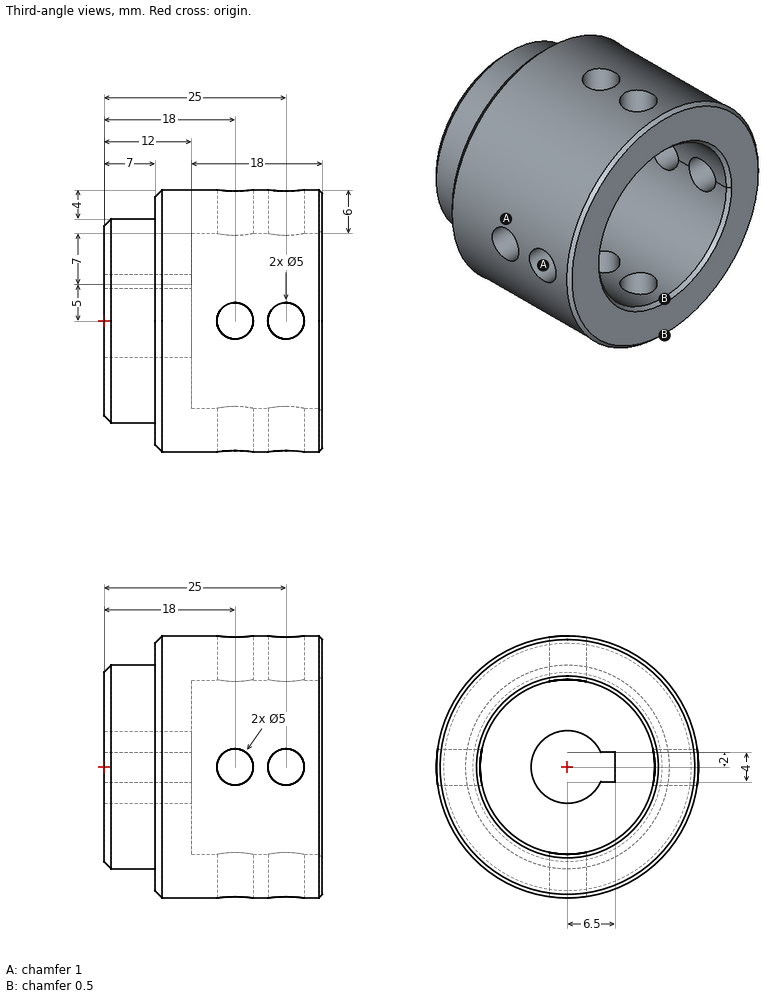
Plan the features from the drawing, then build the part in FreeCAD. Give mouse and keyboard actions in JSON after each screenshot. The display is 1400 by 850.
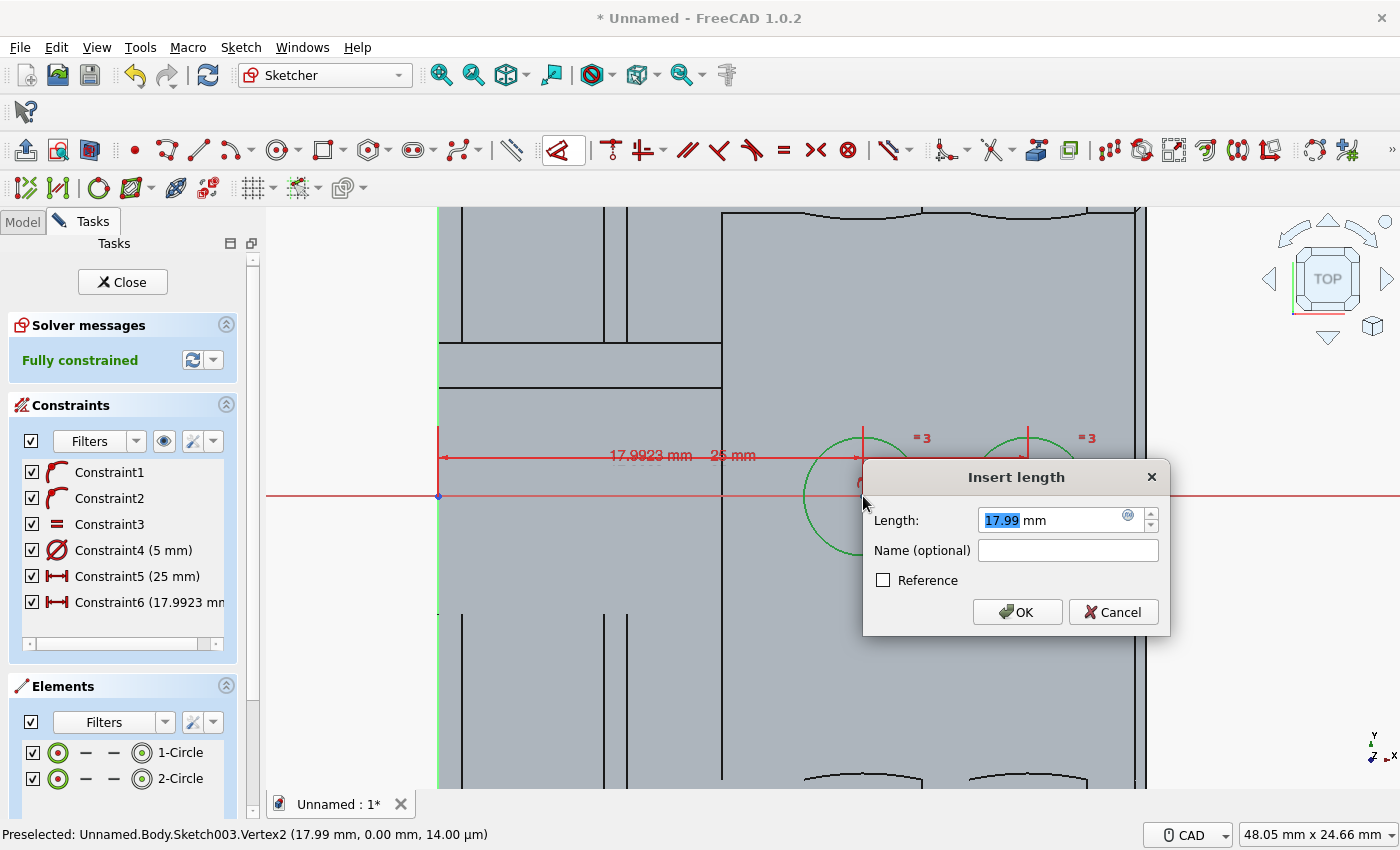
{"action": "type", "text": "18"}
{"action": "key", "text": "Return"}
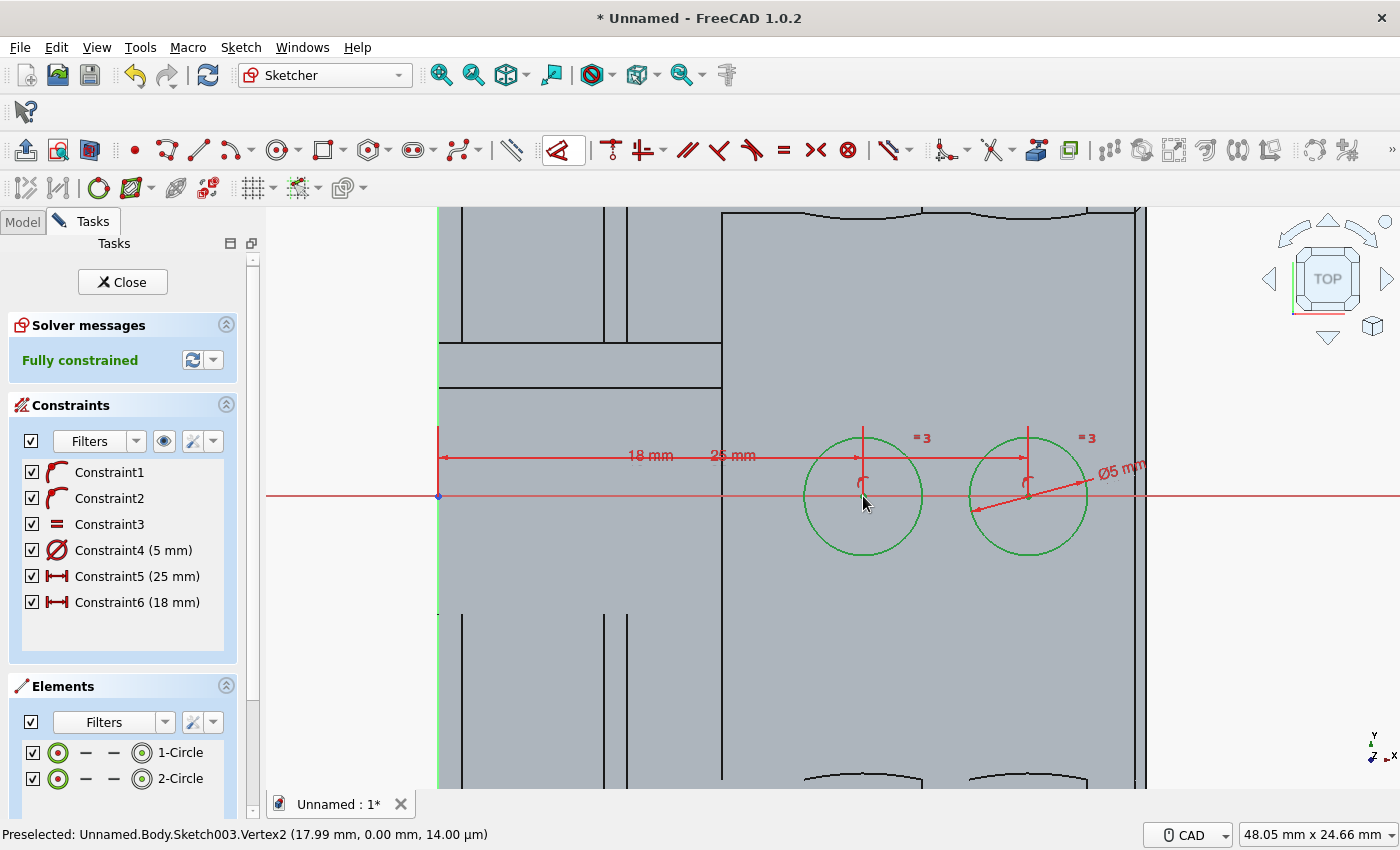
{"action": "left_click", "coordinate": [123, 282]}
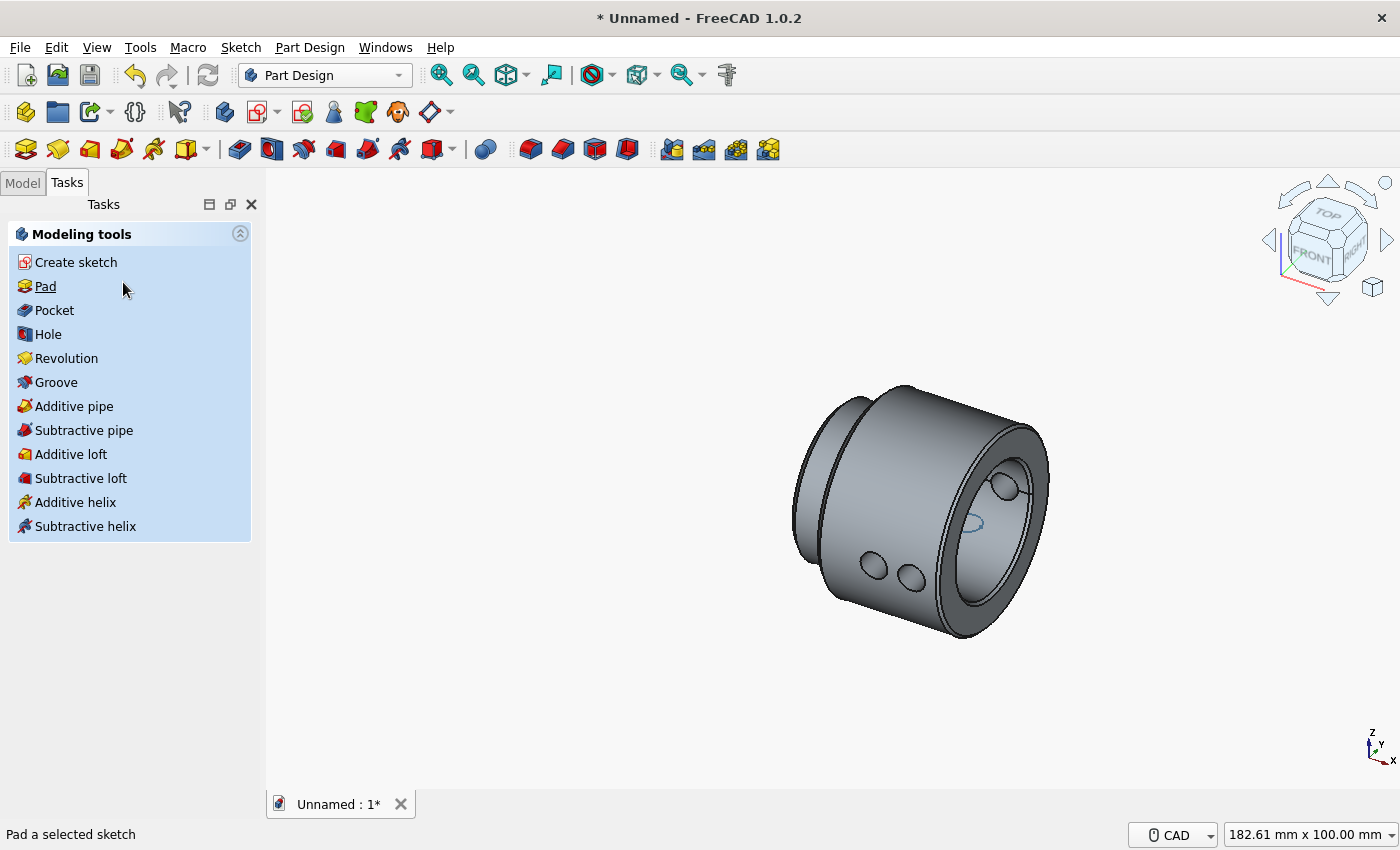
{"action": "left_click", "coordinate": [240, 150]}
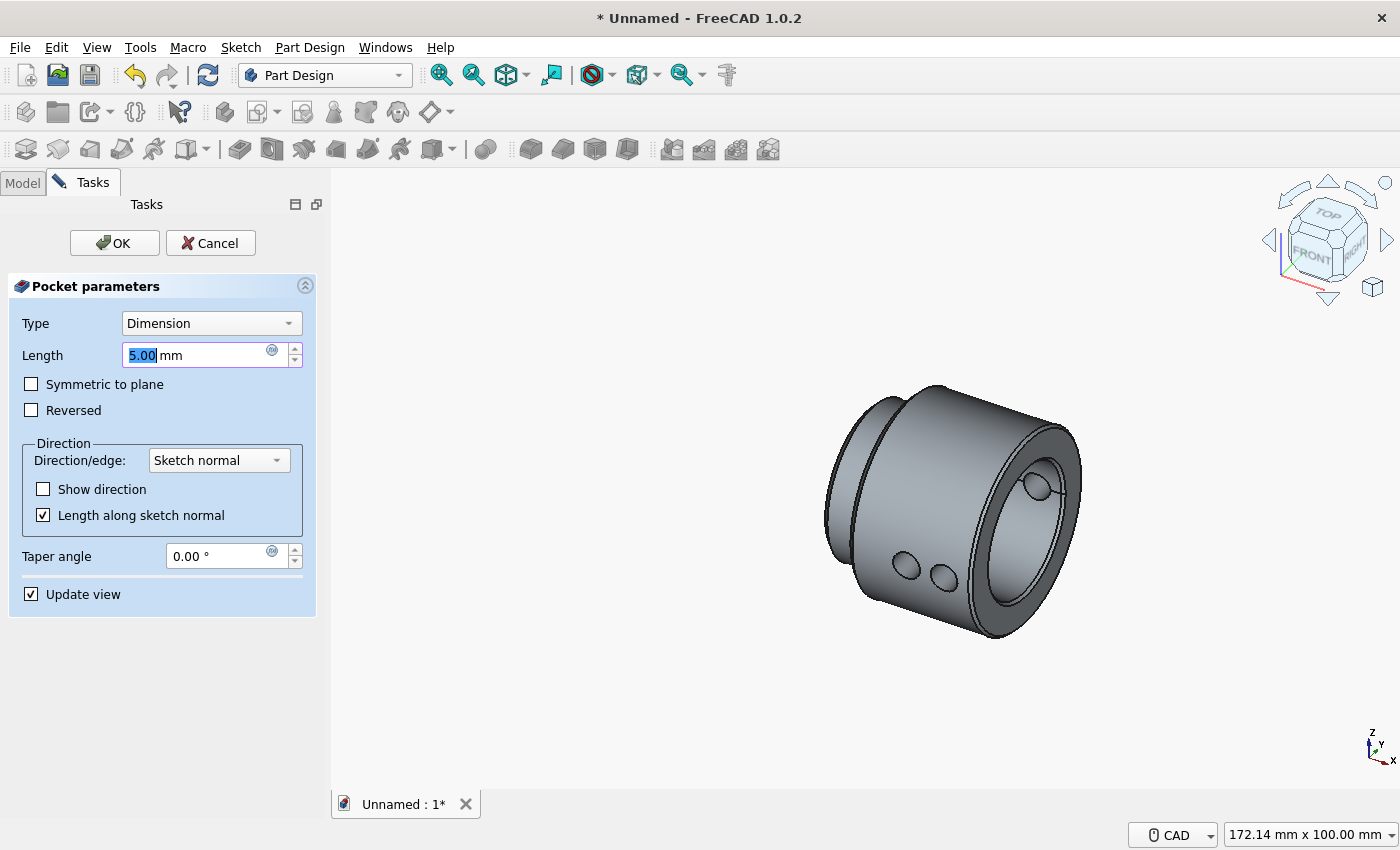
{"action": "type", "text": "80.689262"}
{"action": "key", "text": "Tab"}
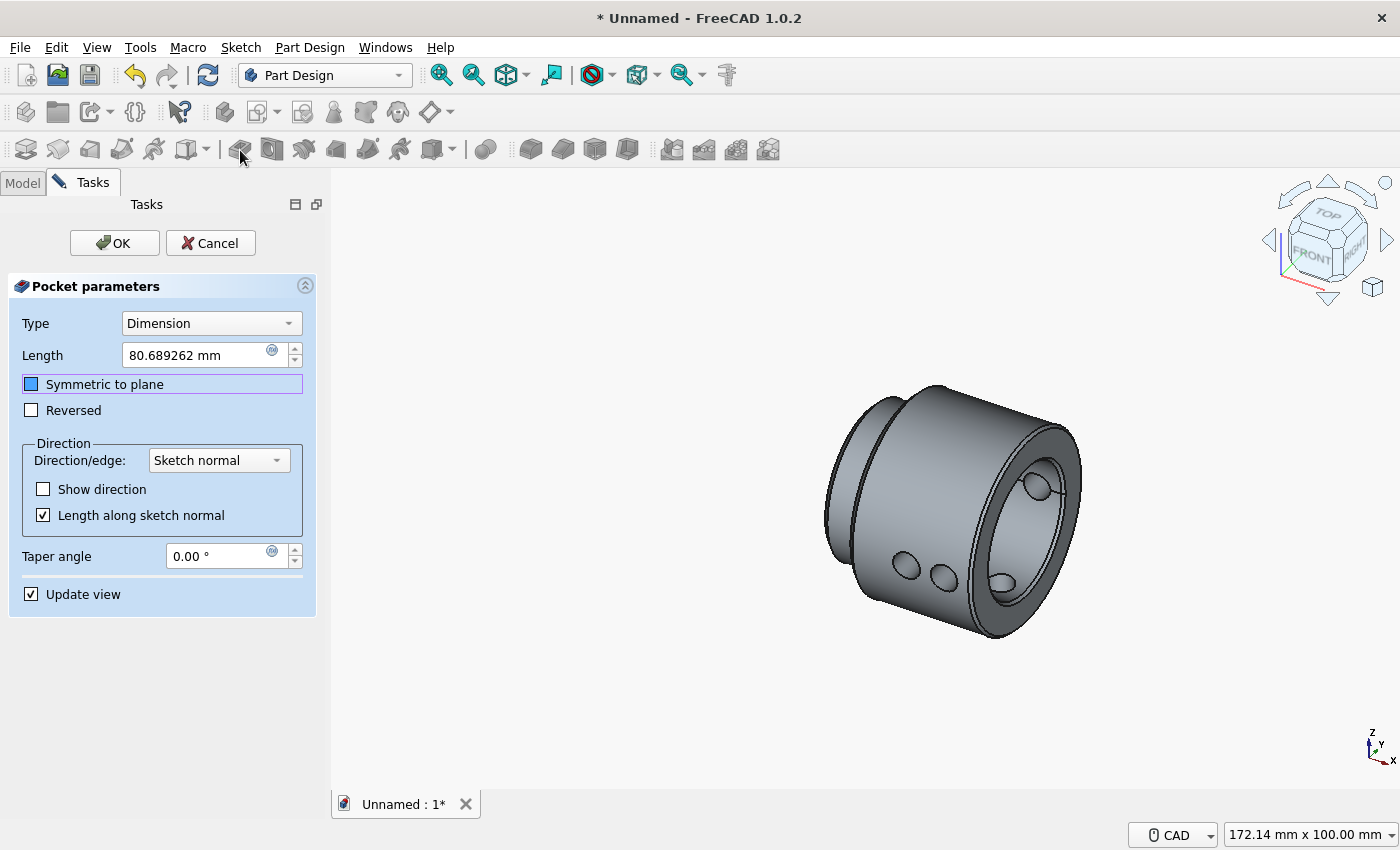
{"action": "left_click", "coordinate": [30, 384]}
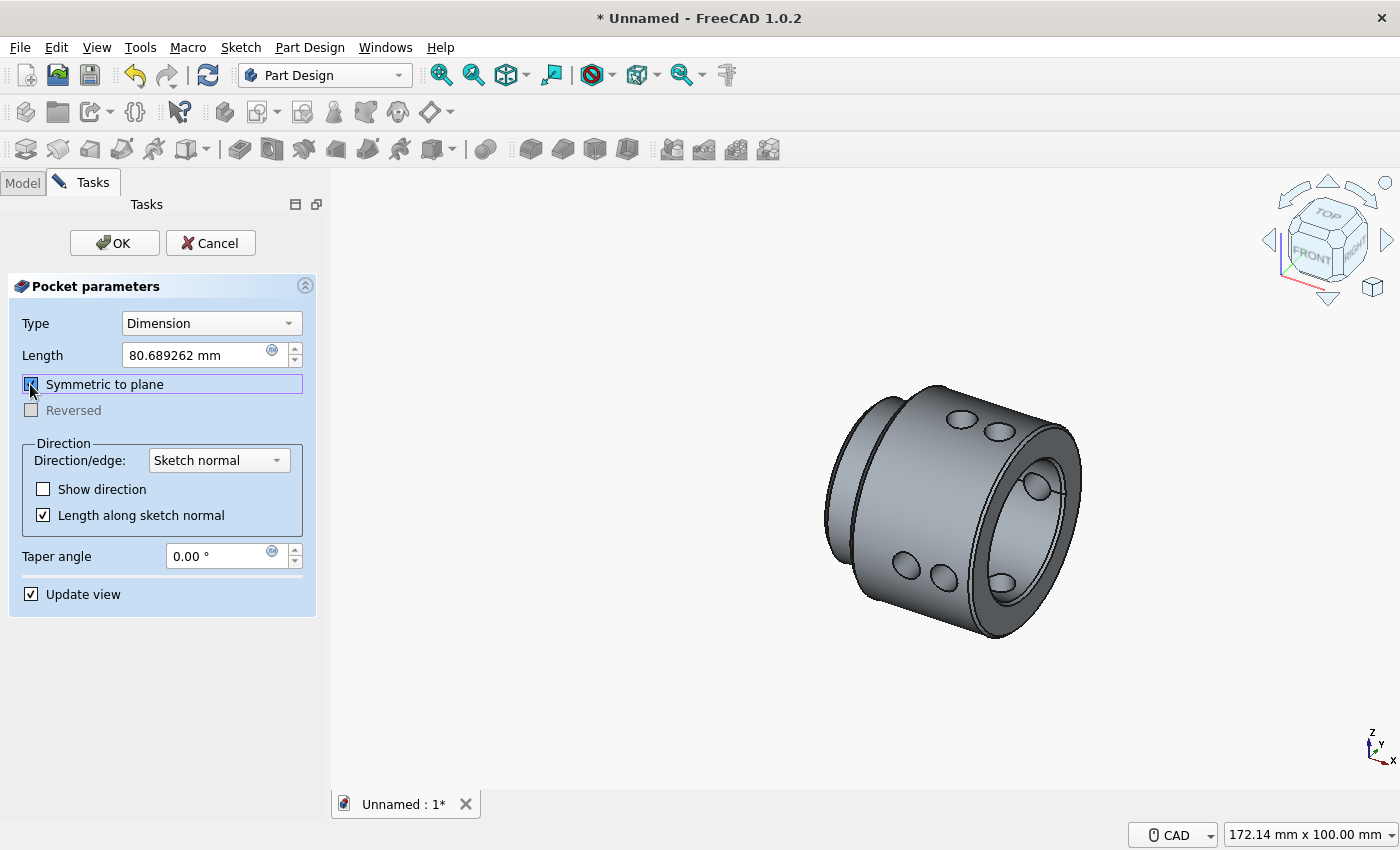
{"action": "left_click", "coordinate": [115, 243]}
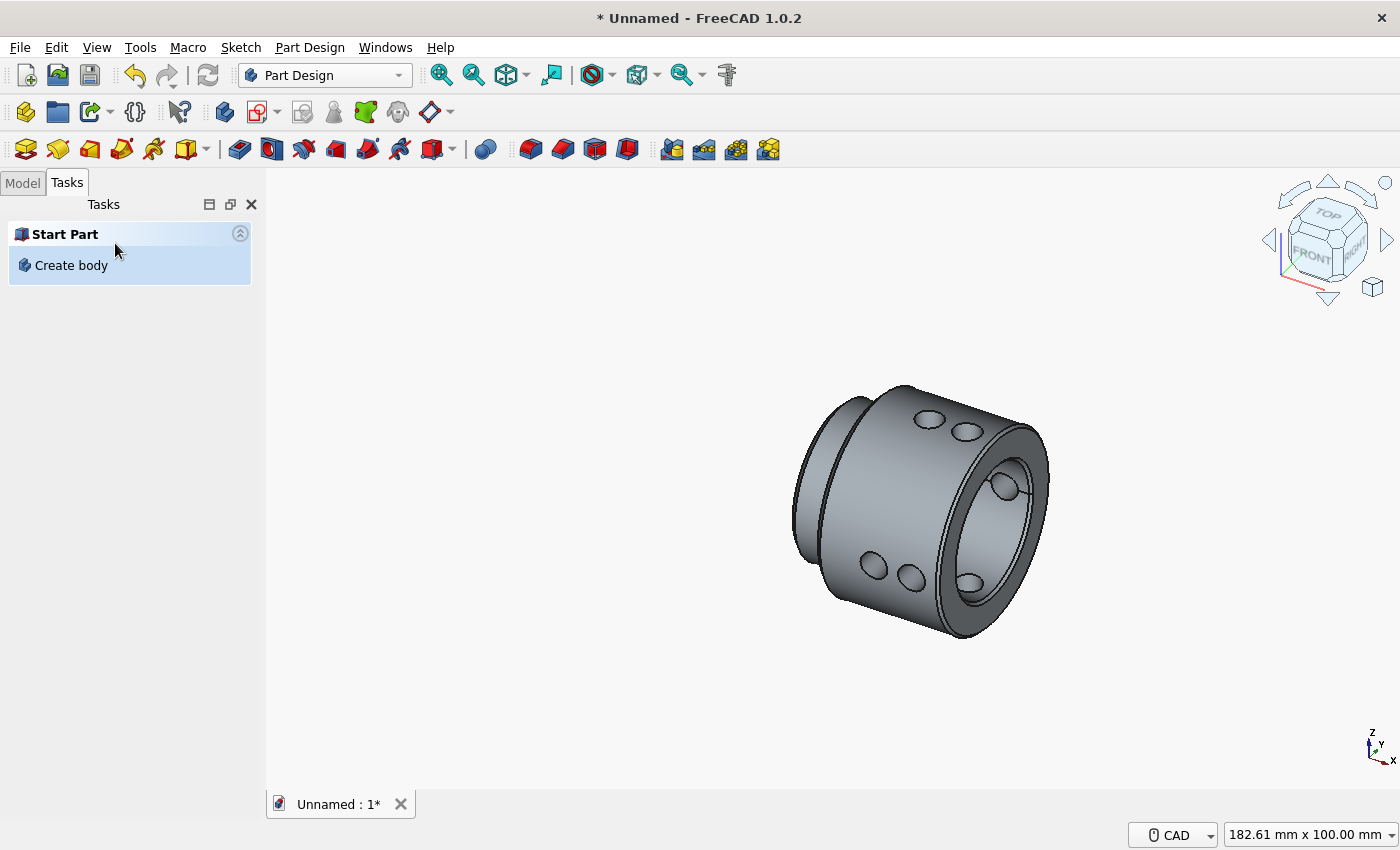
{"action": "key", "text": "0"}